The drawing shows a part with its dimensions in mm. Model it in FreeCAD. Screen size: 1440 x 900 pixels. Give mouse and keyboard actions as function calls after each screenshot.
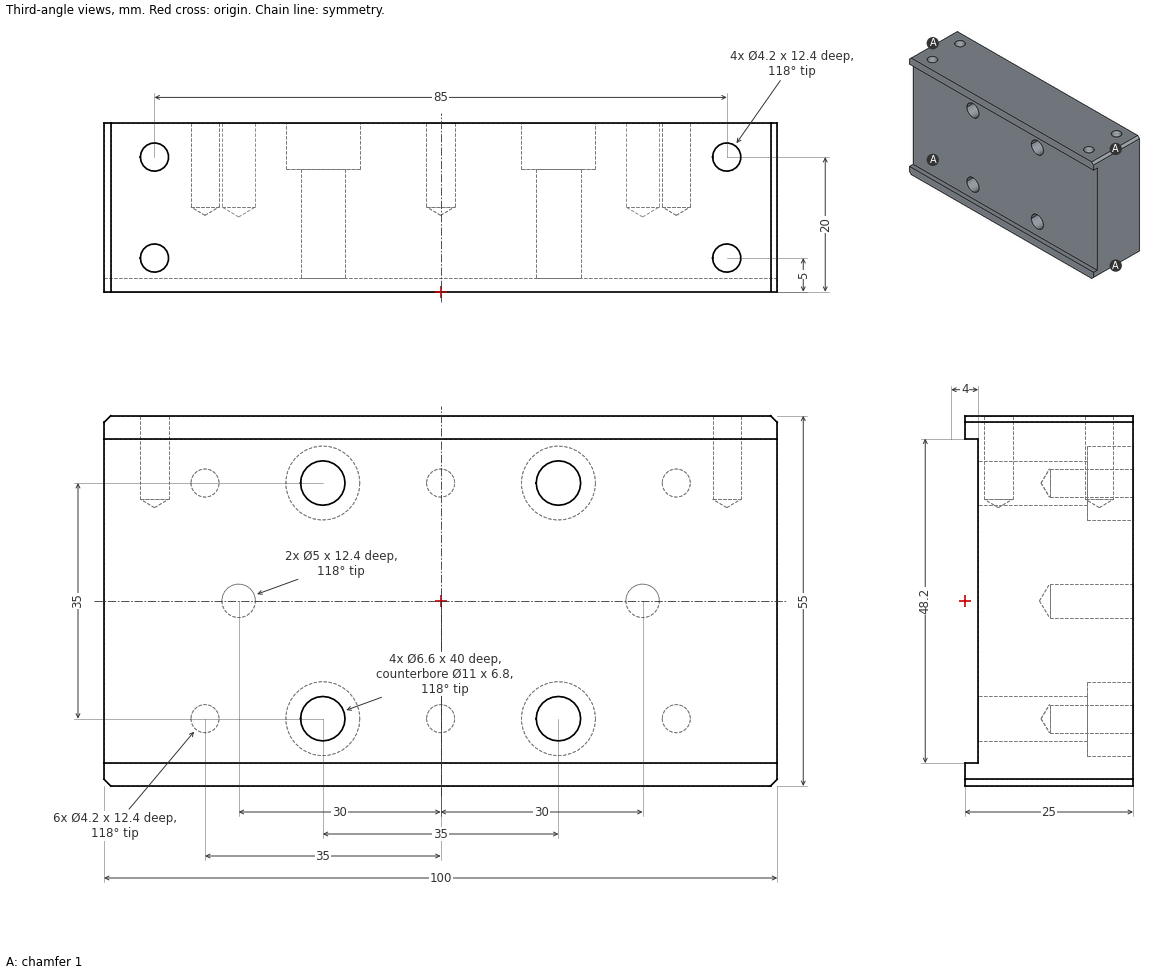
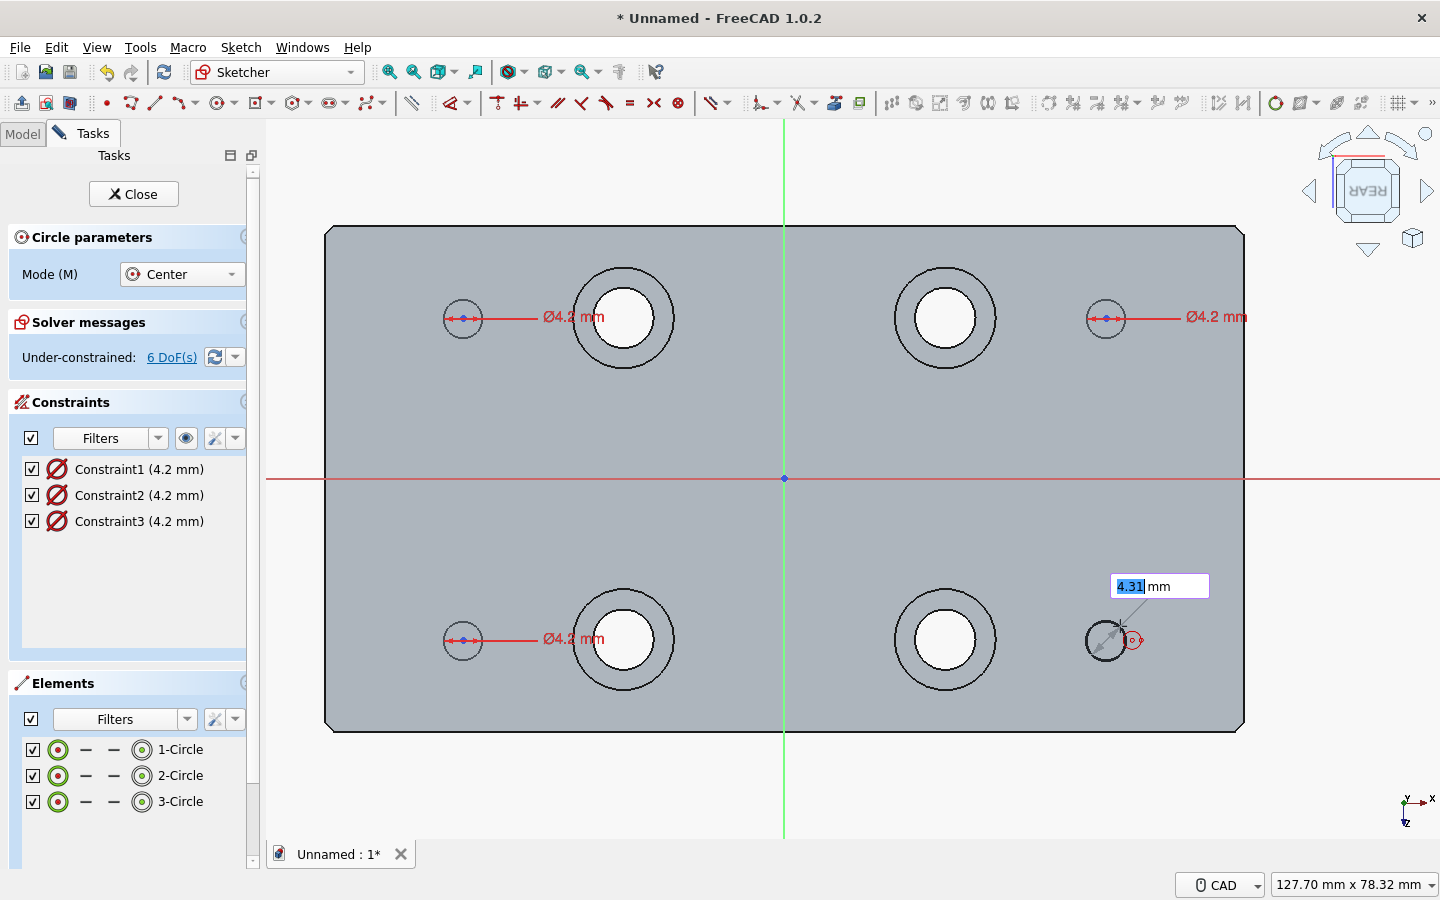
text(4.2)
key(Return)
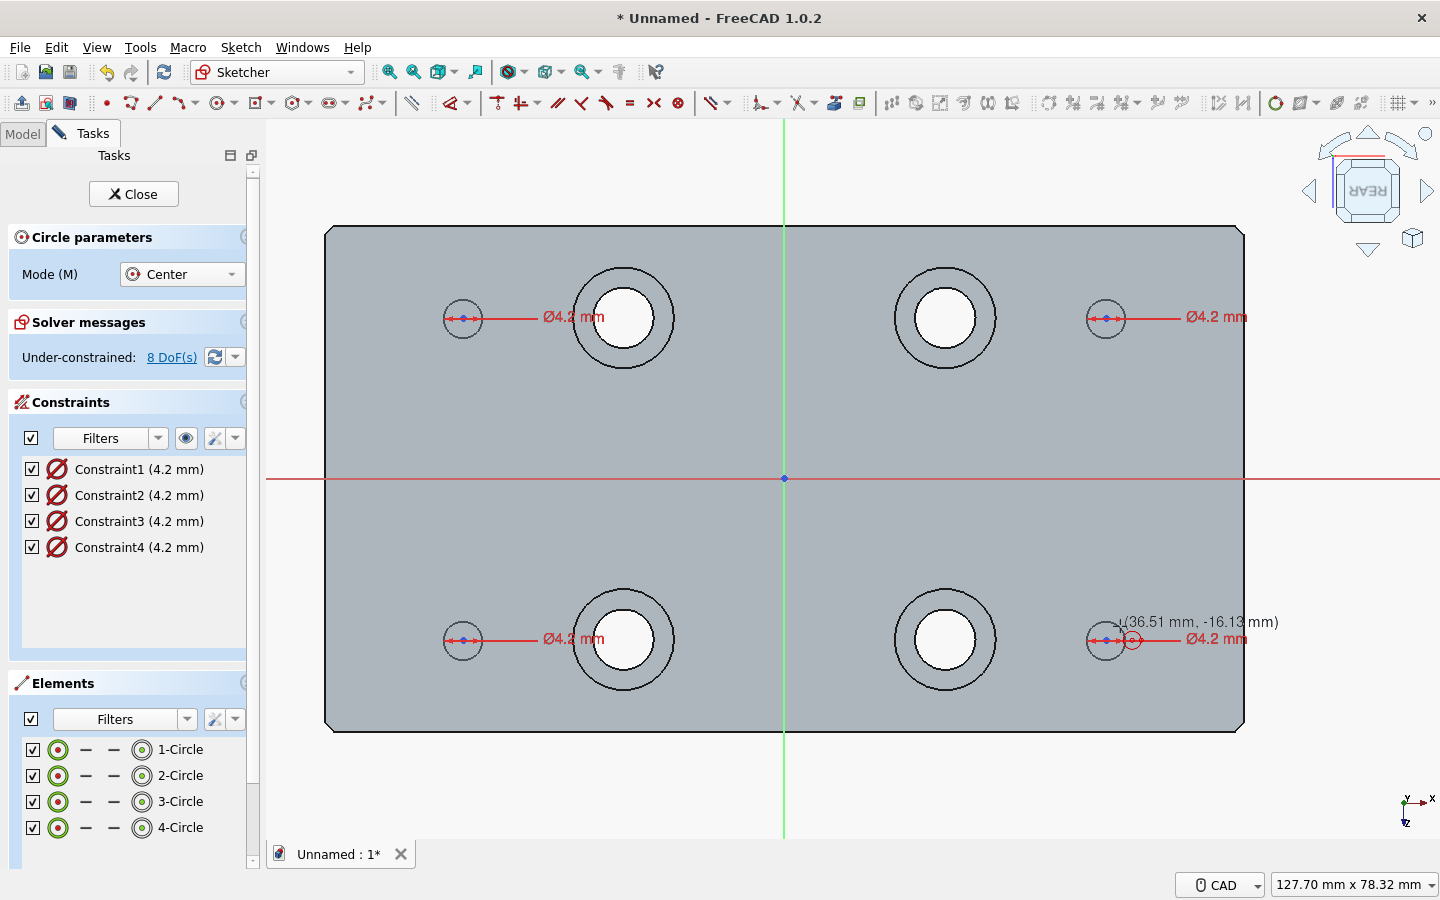
click(784, 318)
move(802, 311)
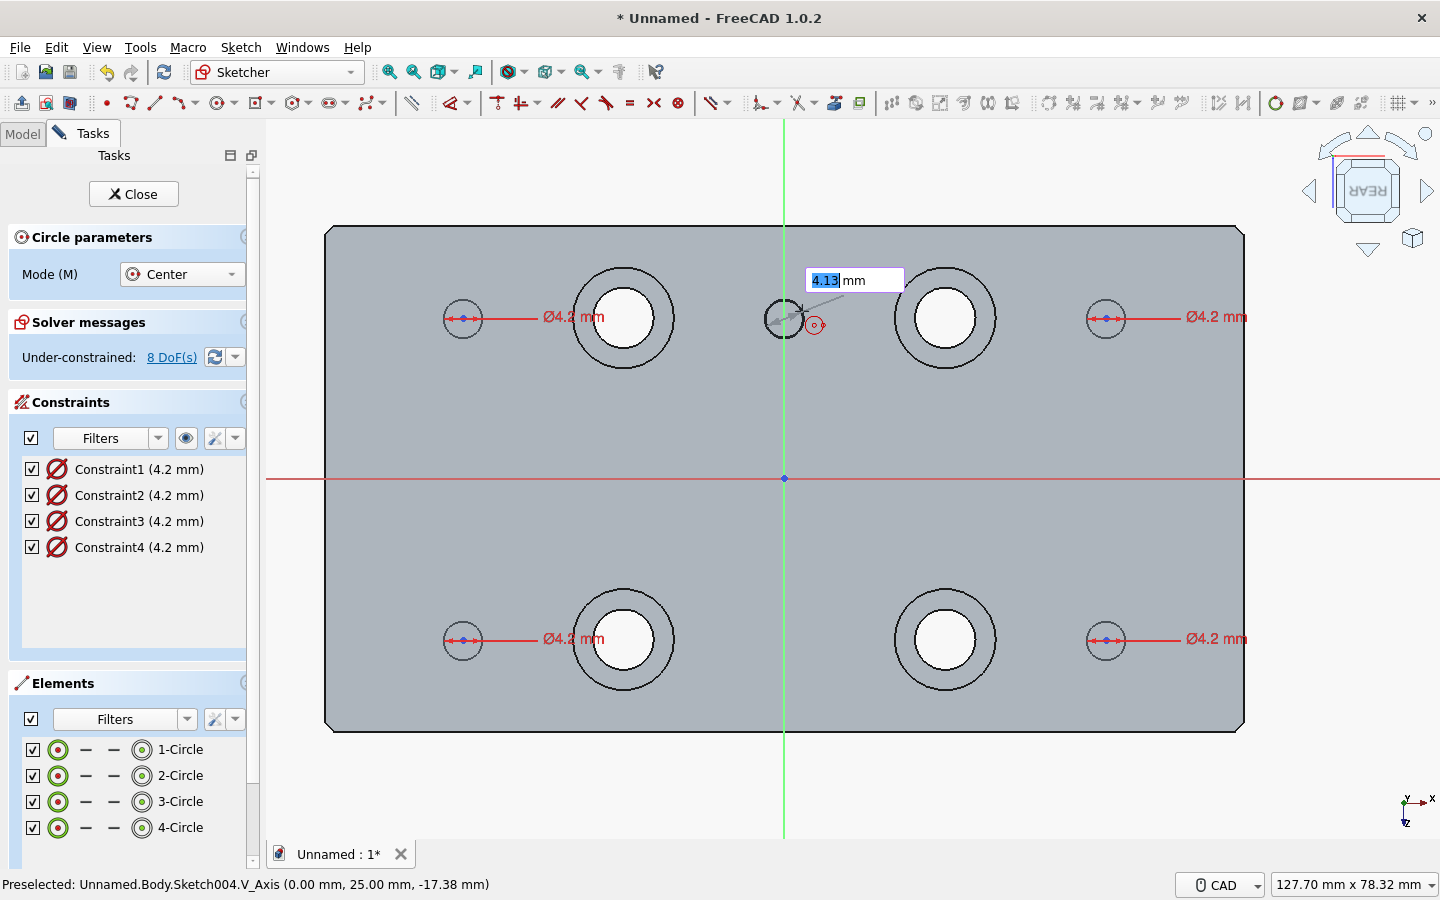
text(4.2)
key(Return)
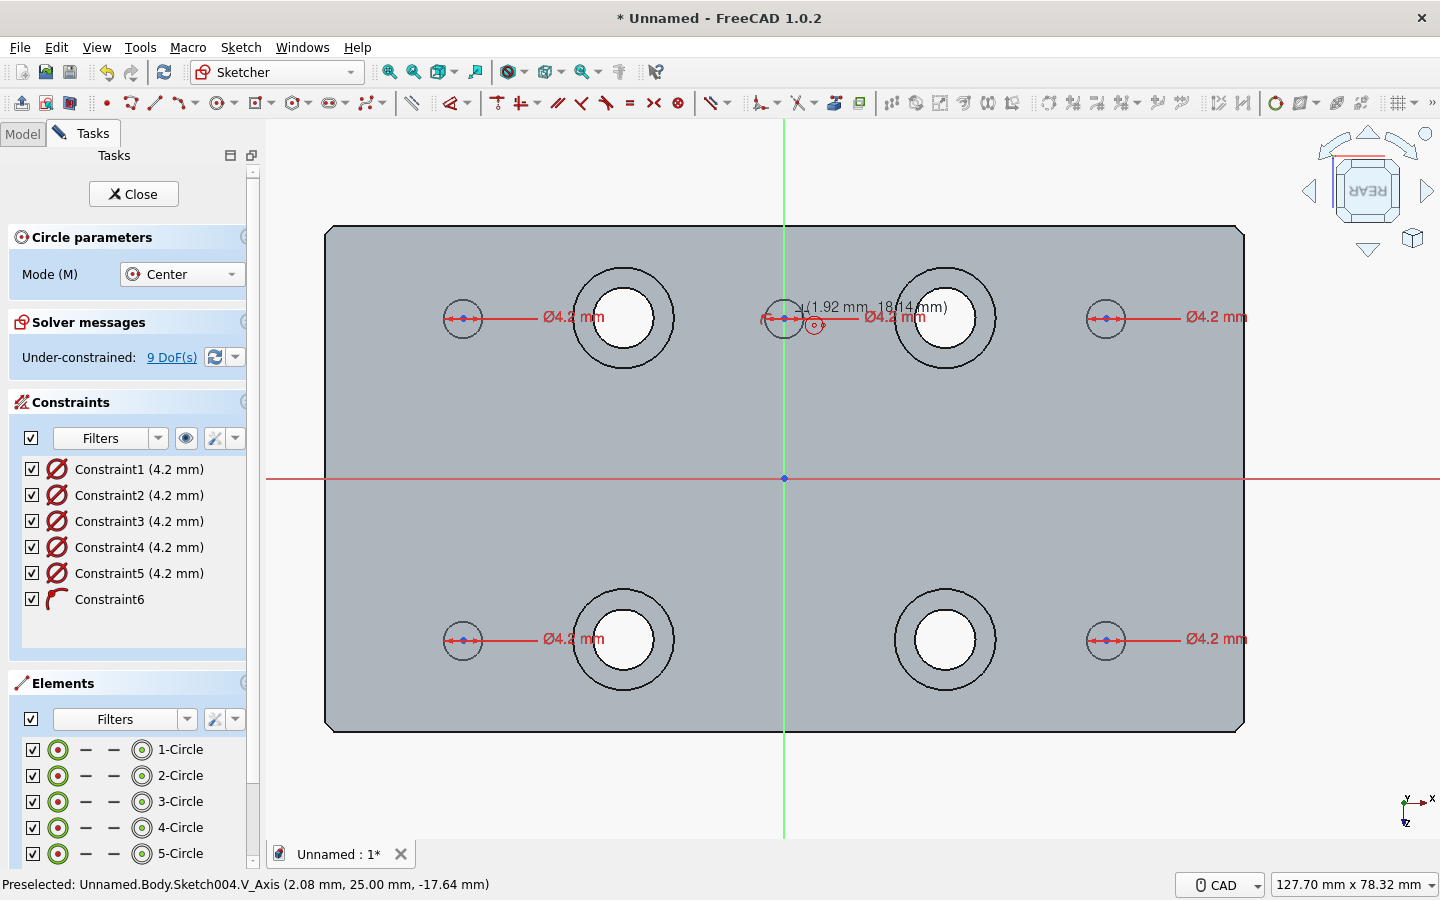
click(784, 640)
move(802, 633)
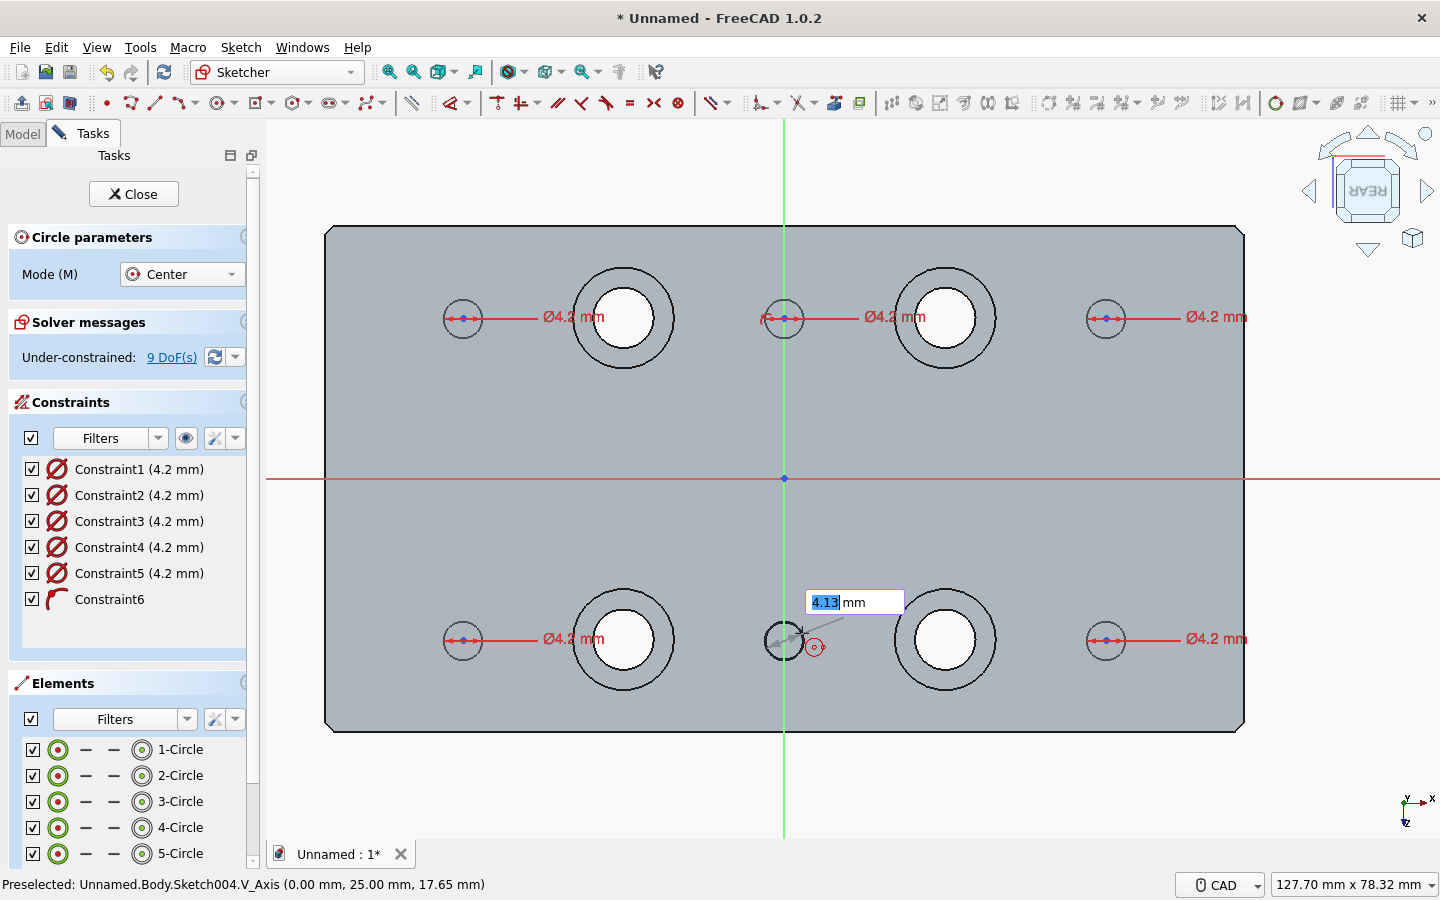
text(4.2)
key(Return)
key(Escape)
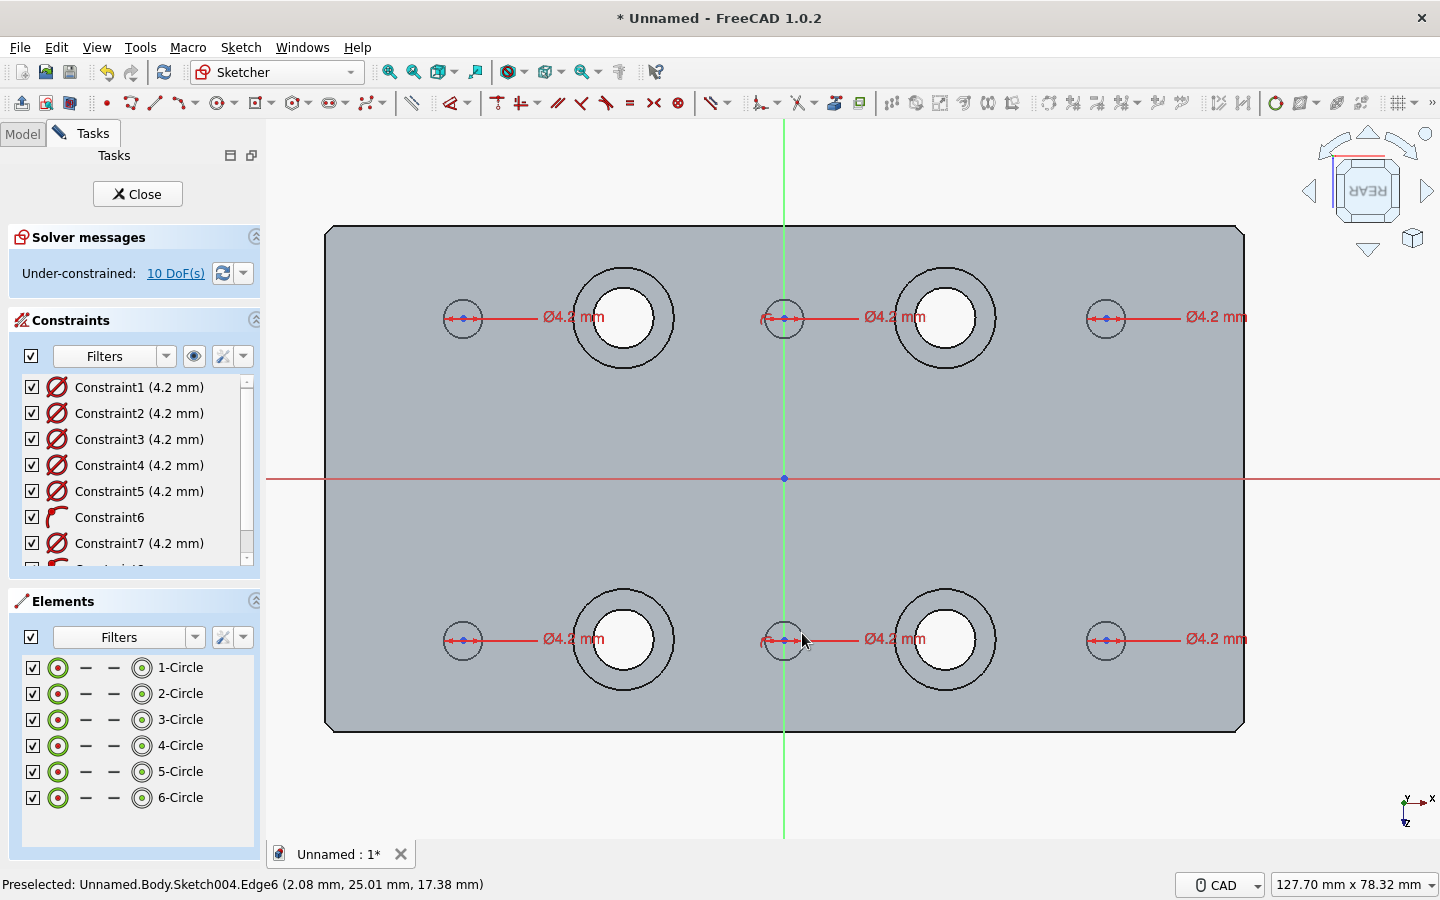
click(463, 319)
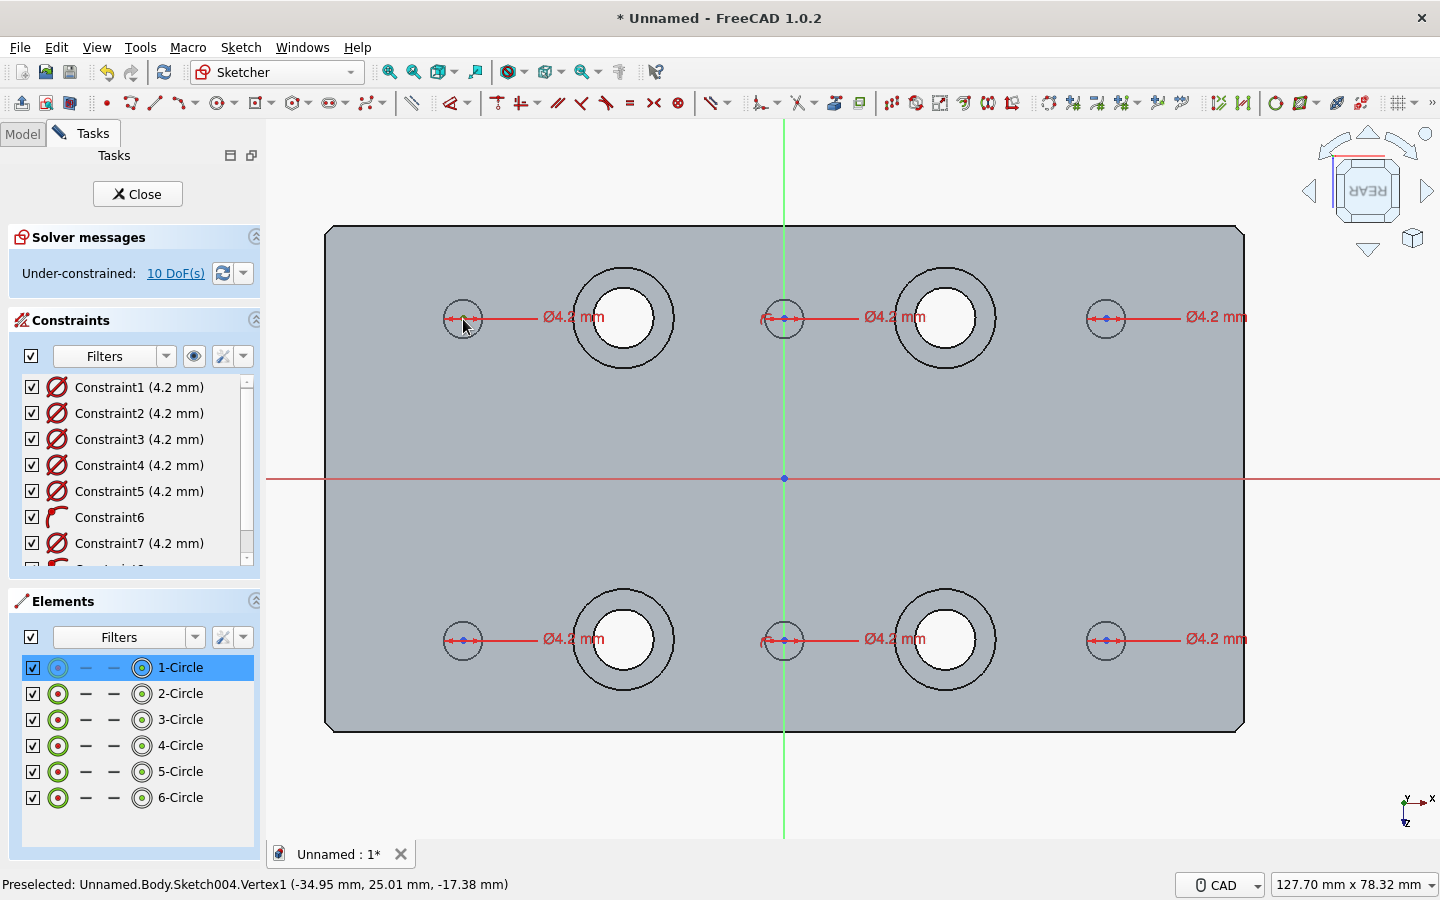
click(463, 641)